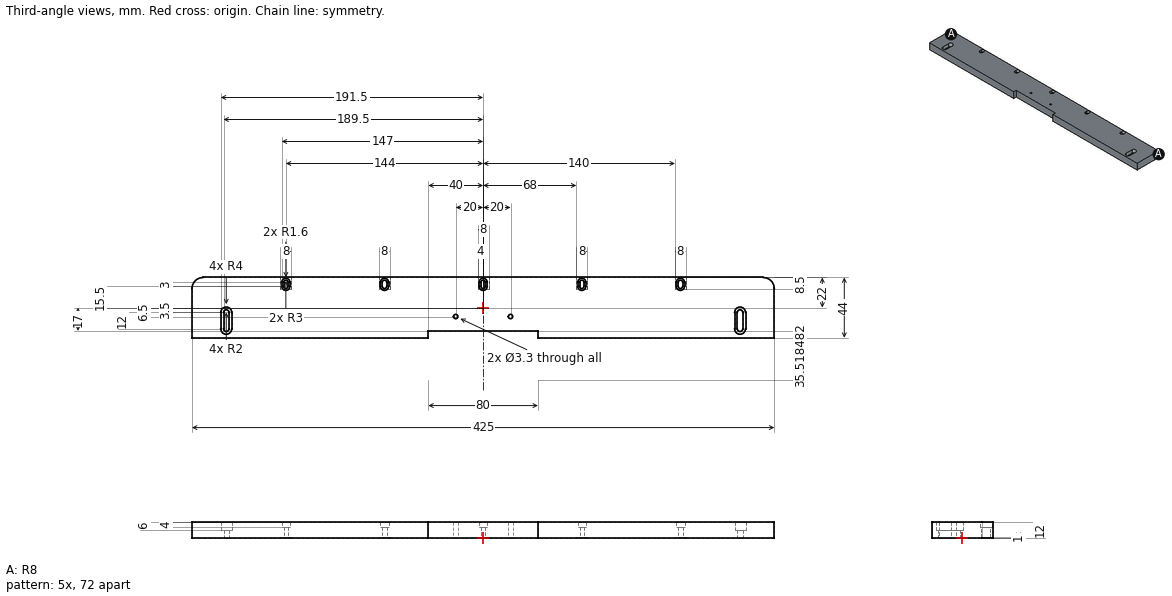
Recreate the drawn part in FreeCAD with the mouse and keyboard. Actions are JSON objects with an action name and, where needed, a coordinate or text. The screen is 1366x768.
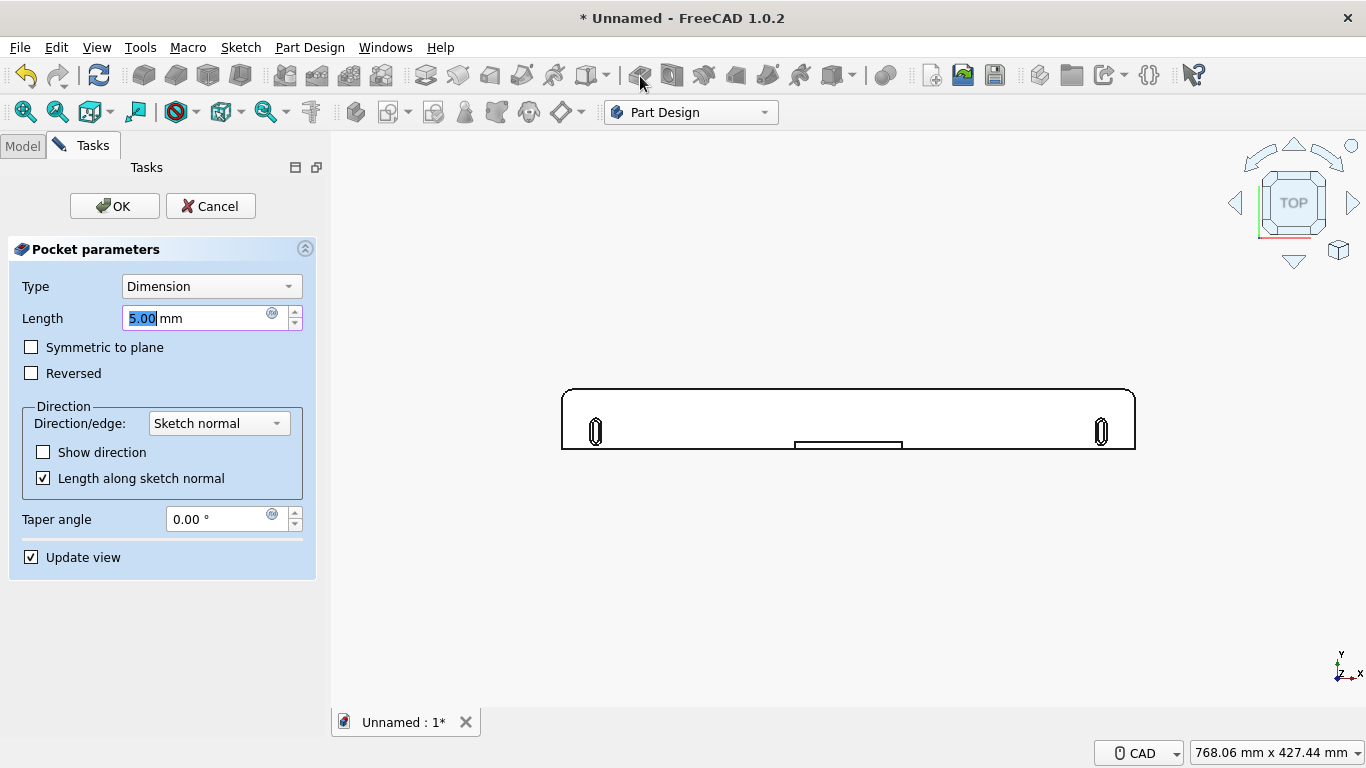
{"action": "left_click", "coordinate": [212, 286]}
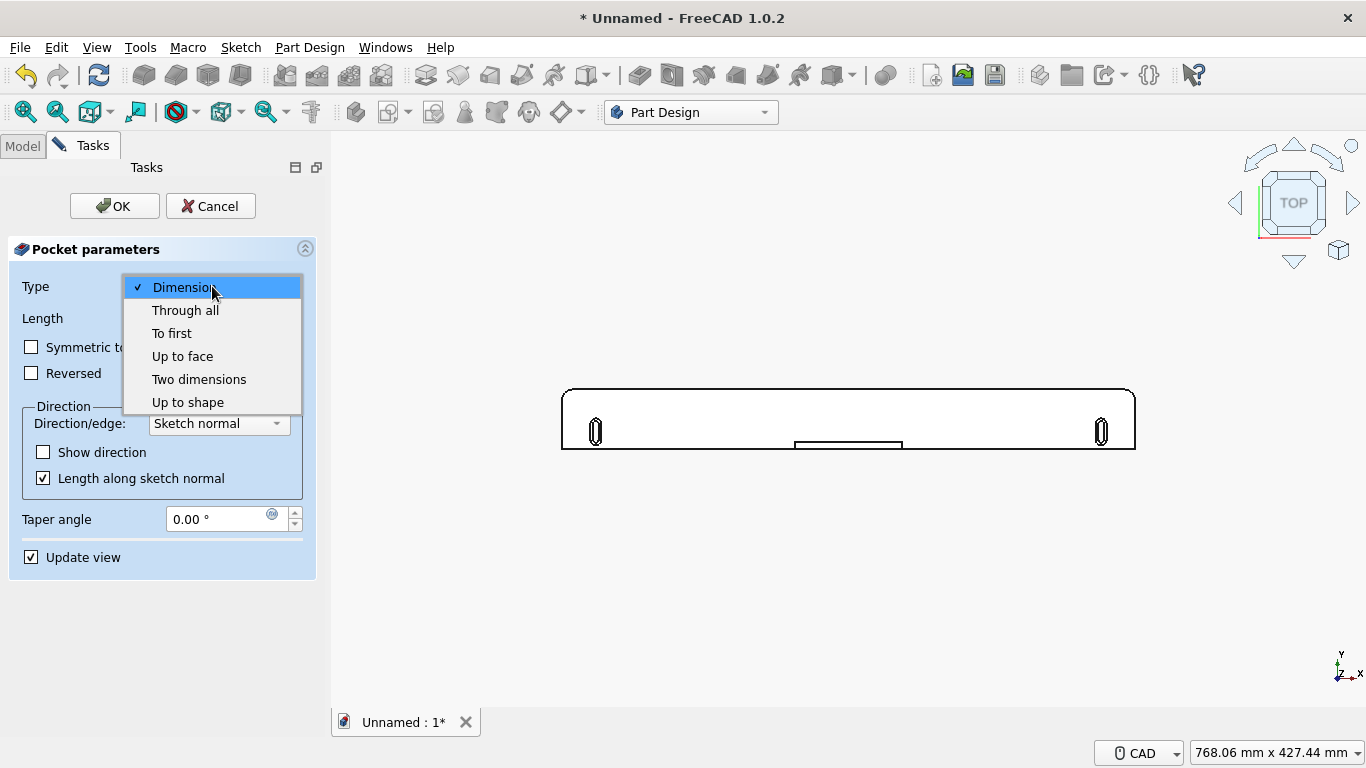
{"action": "left_click", "coordinate": [212, 310]}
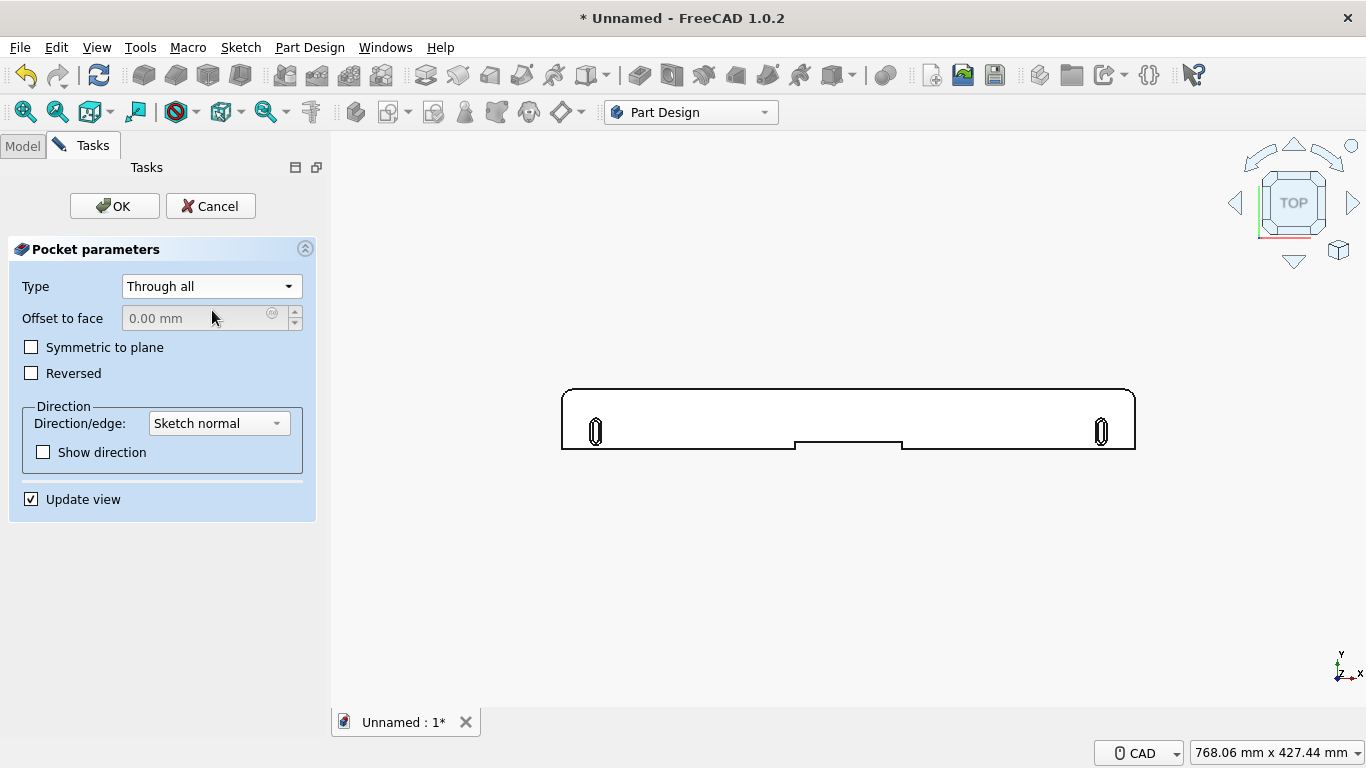
{"action": "left_click", "coordinate": [115, 206]}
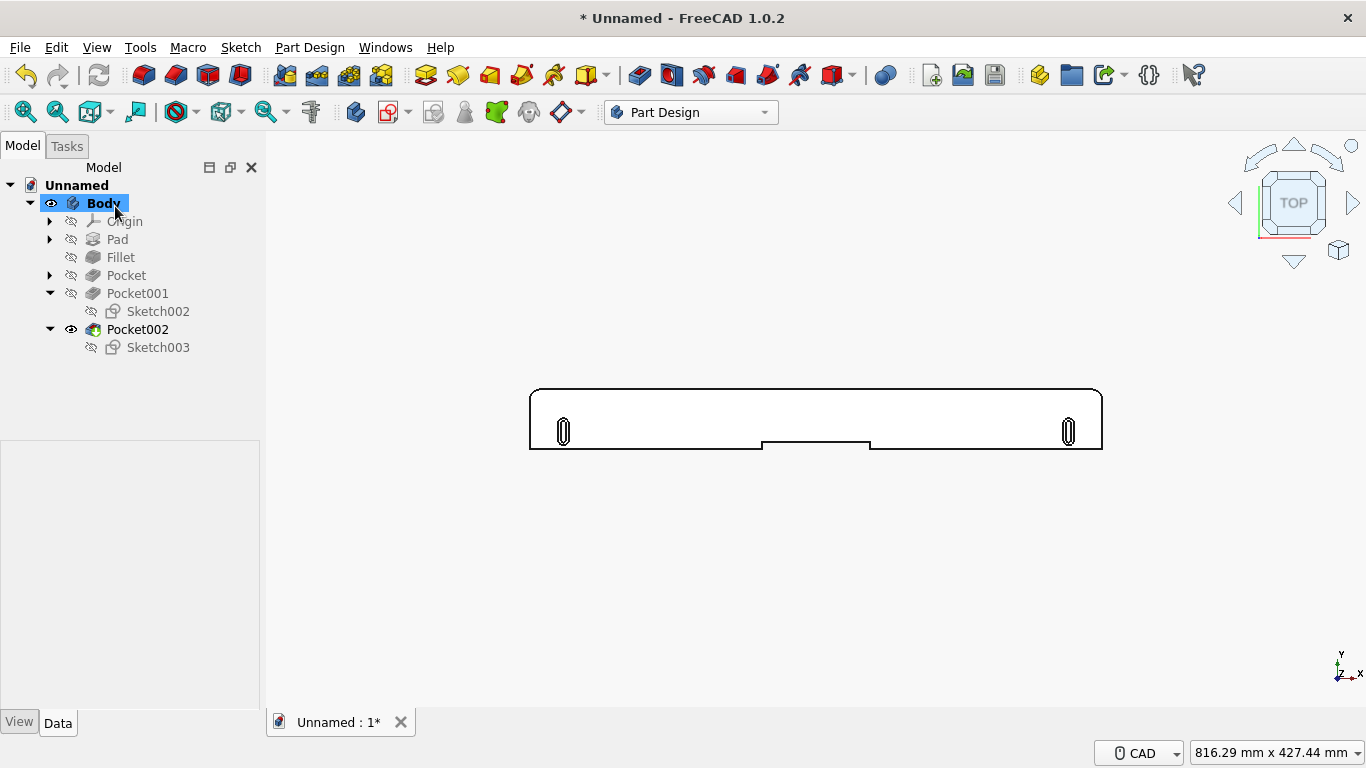
{"action": "left_click", "coordinate": [388, 112]}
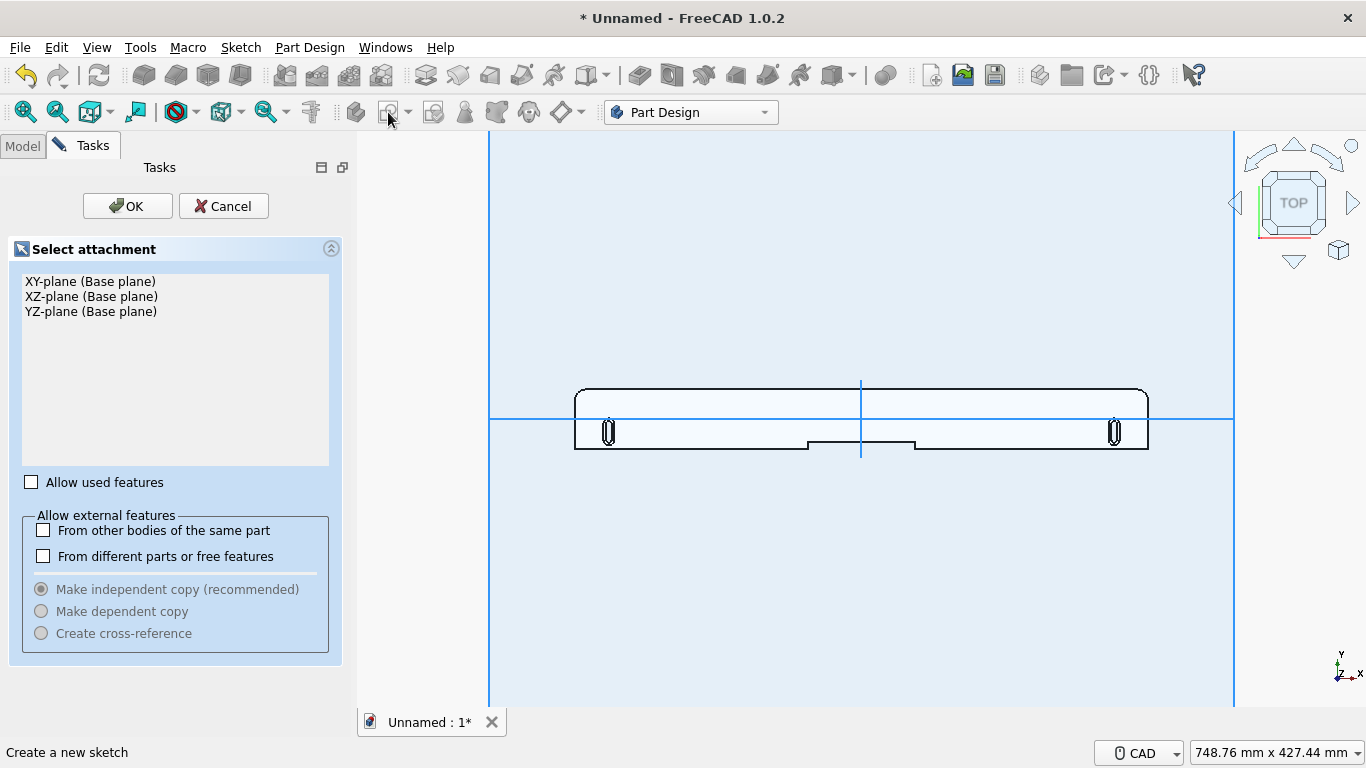
{"action": "left_click", "coordinate": [82, 282]}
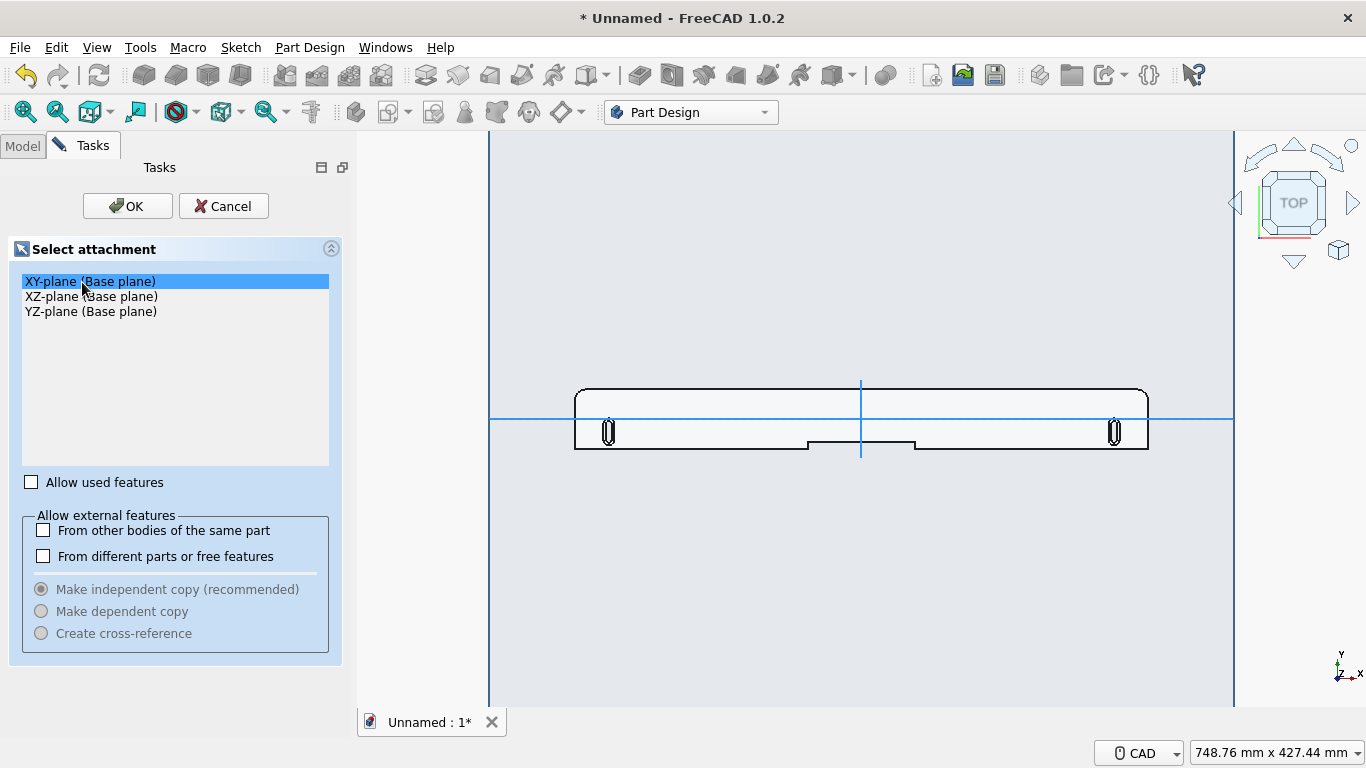
{"action": "left_click", "coordinate": [128, 206]}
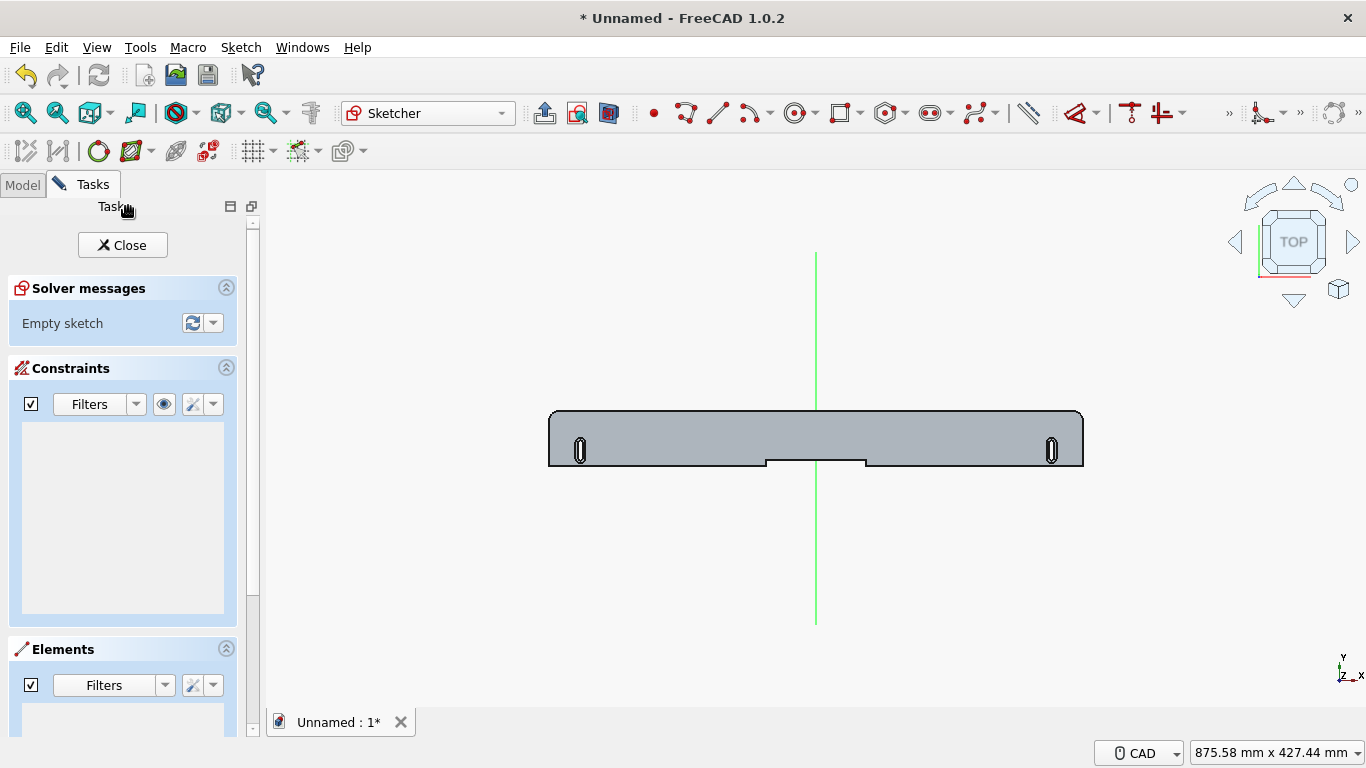
{"action": "key", "text": "q s"}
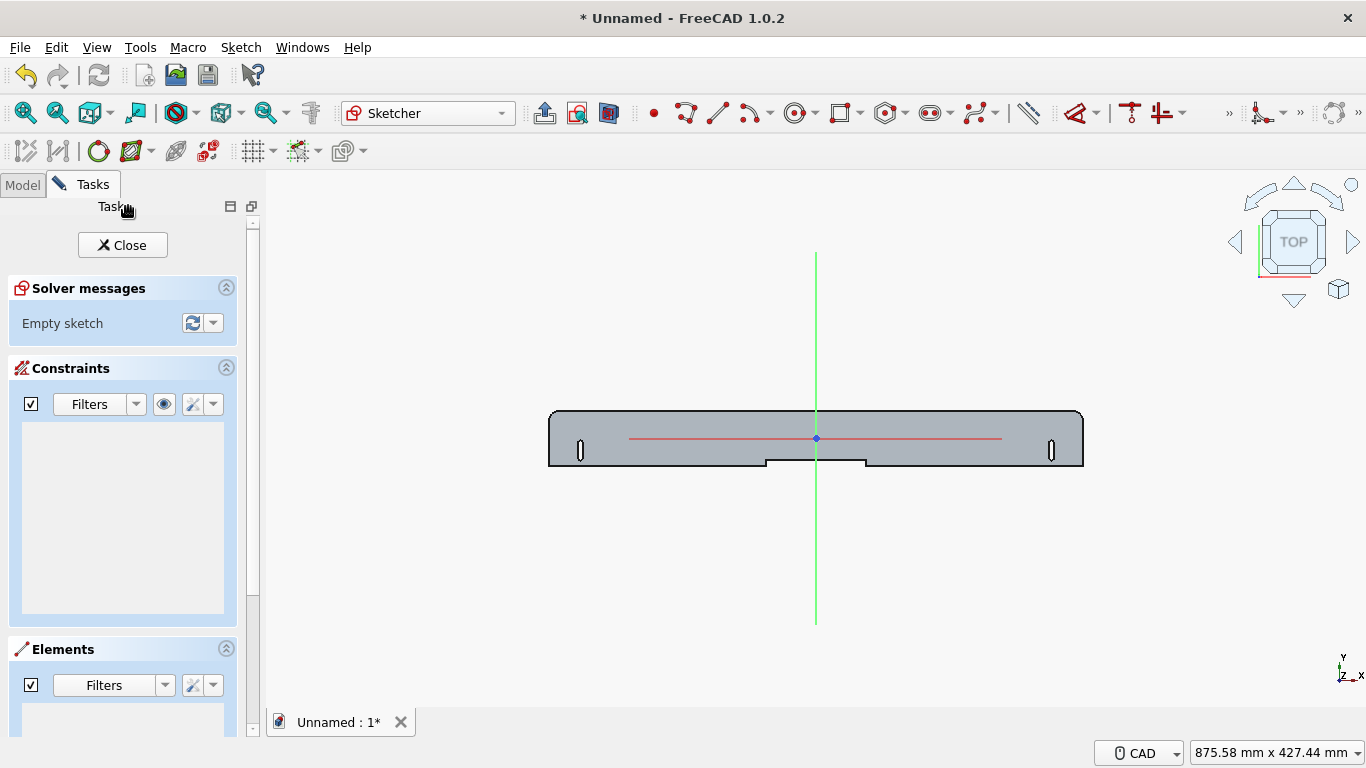
{"action": "scroll", "coordinate": [899, 408], "scroll_direction": "up", "scroll_amount": 3}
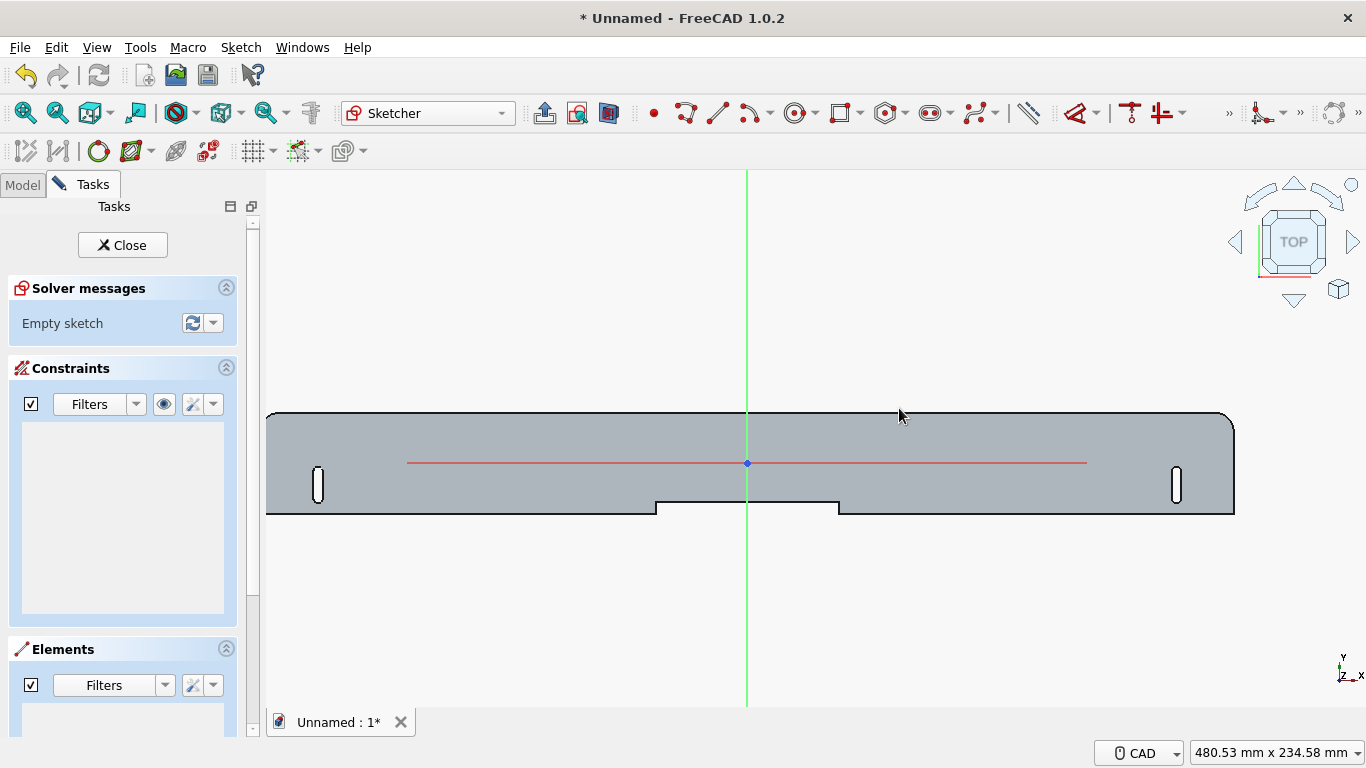
{"action": "left_click", "coordinate": [840, 114]}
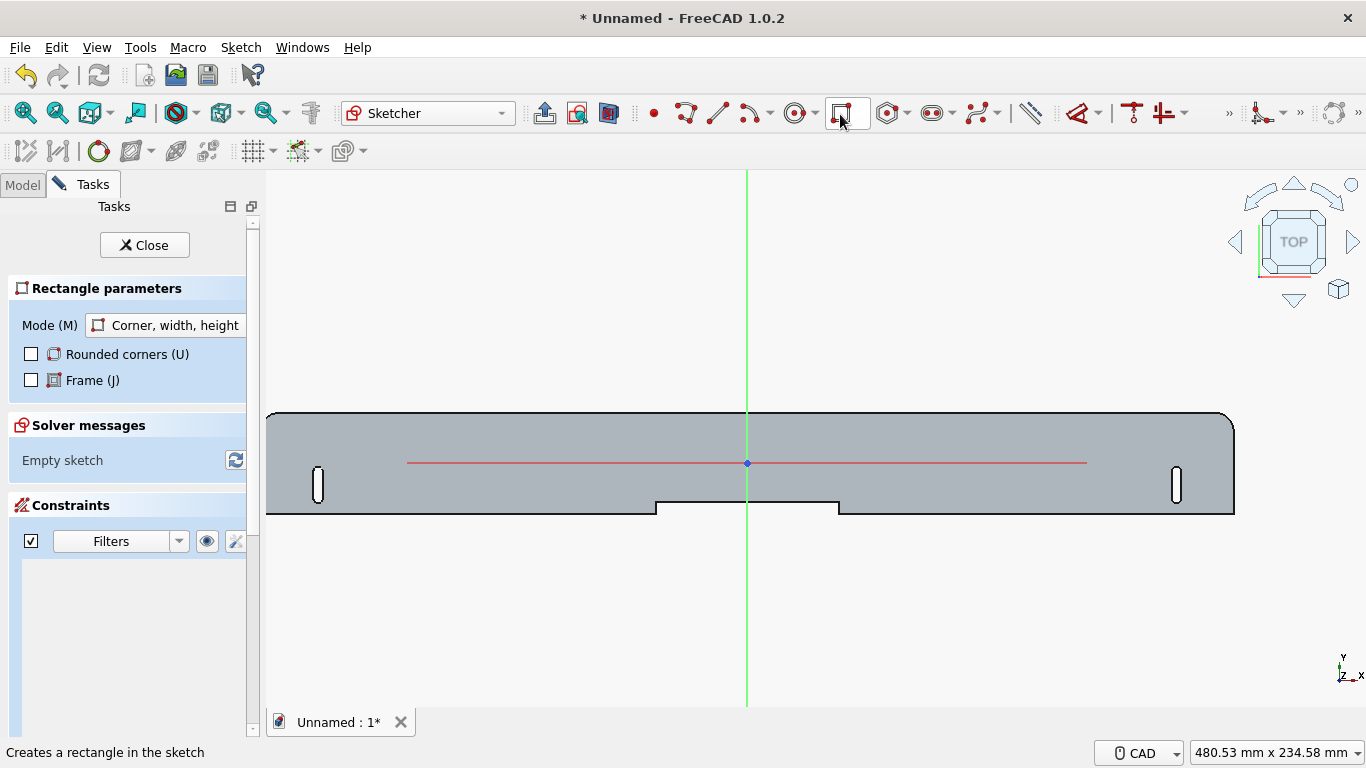
{"action": "left_click", "coordinate": [1068, 413]}
{"action": "mouse_move", "coordinate": [1086, 432]}